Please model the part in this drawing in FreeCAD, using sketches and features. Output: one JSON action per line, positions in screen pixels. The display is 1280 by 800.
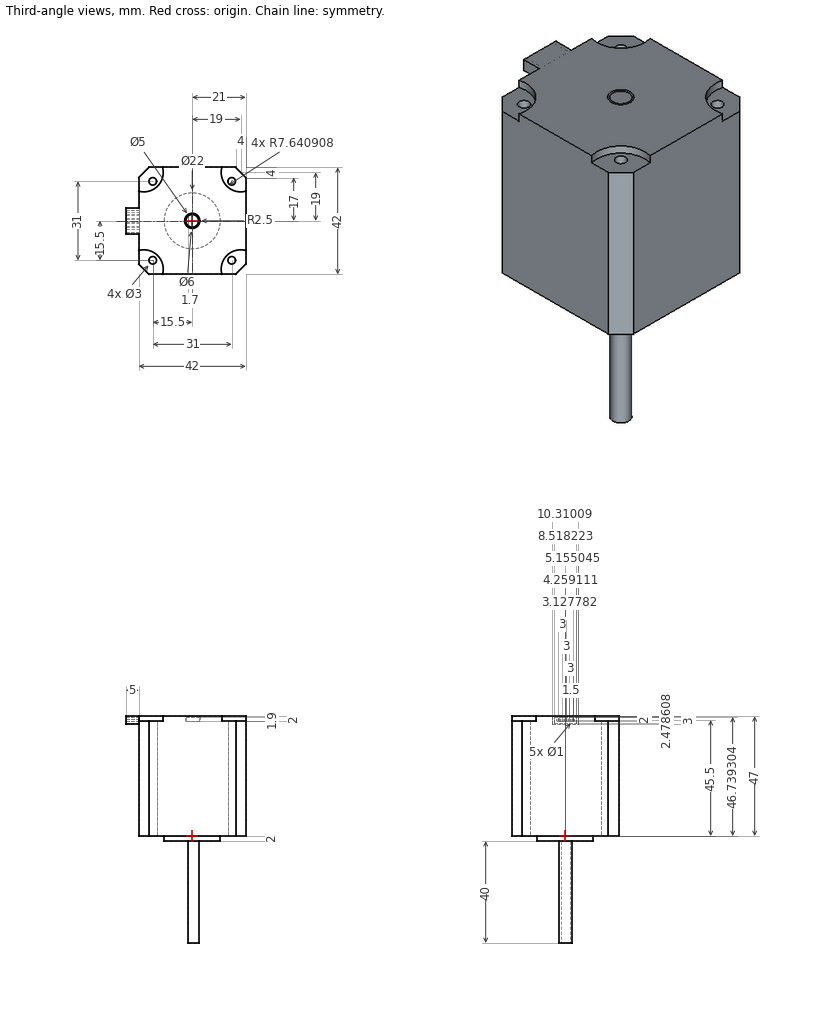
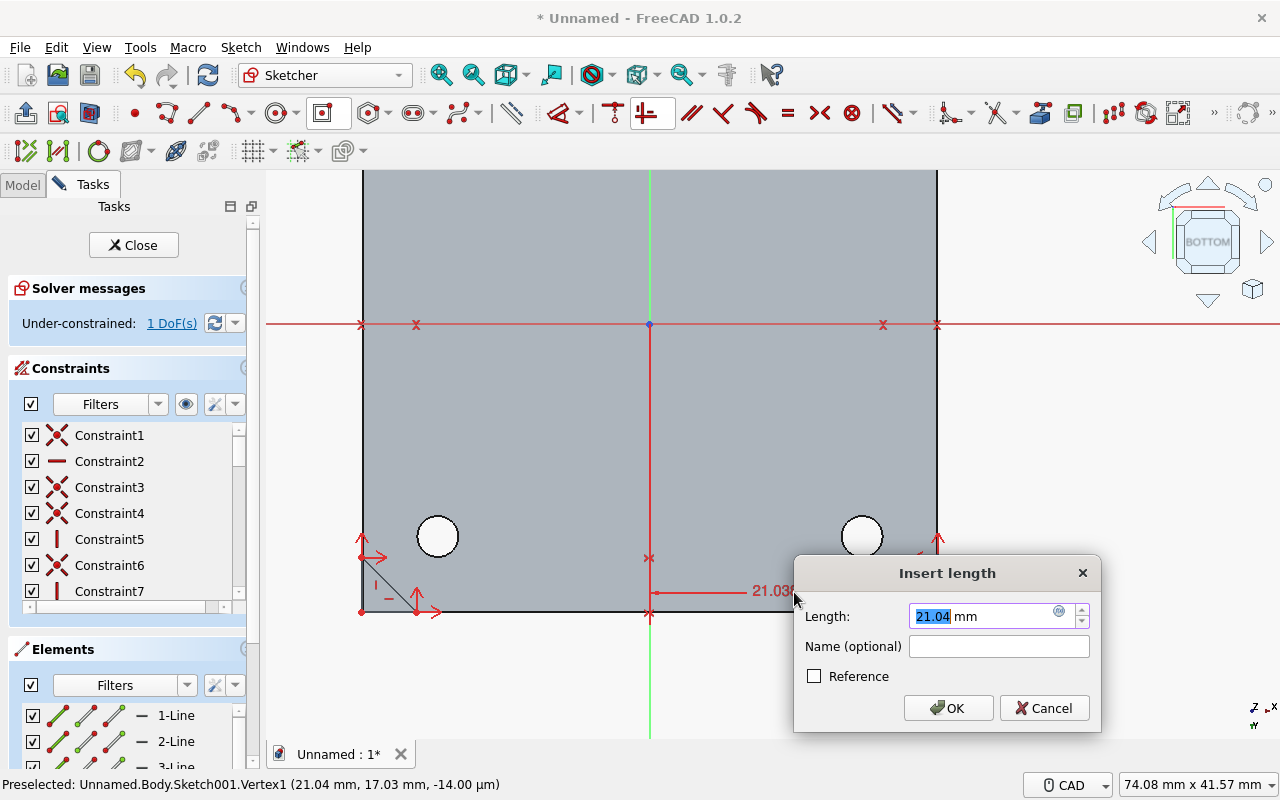
{"action": "type", "text": "21"}
{"action": "key", "text": "Return"}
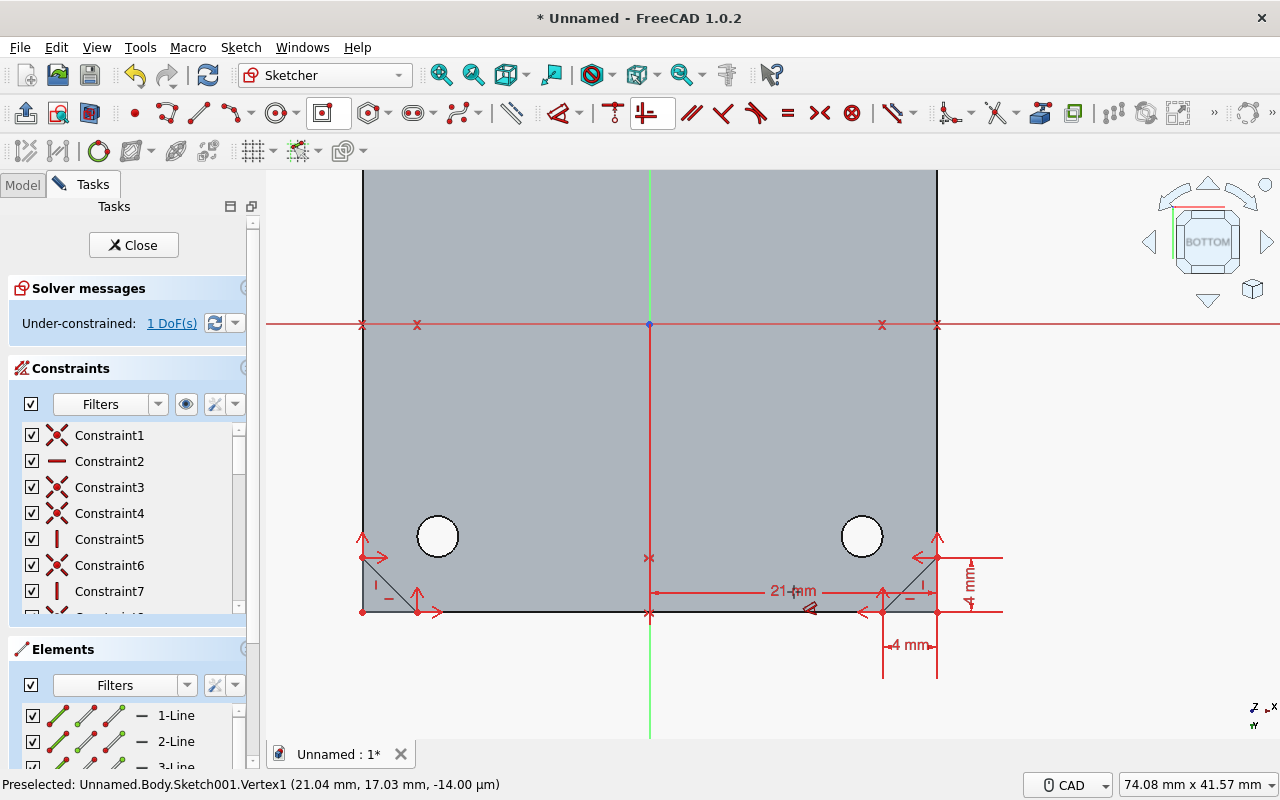
{"action": "left_click", "coordinate": [937, 558]}
{"action": "left_click", "coordinate": [971, 441]}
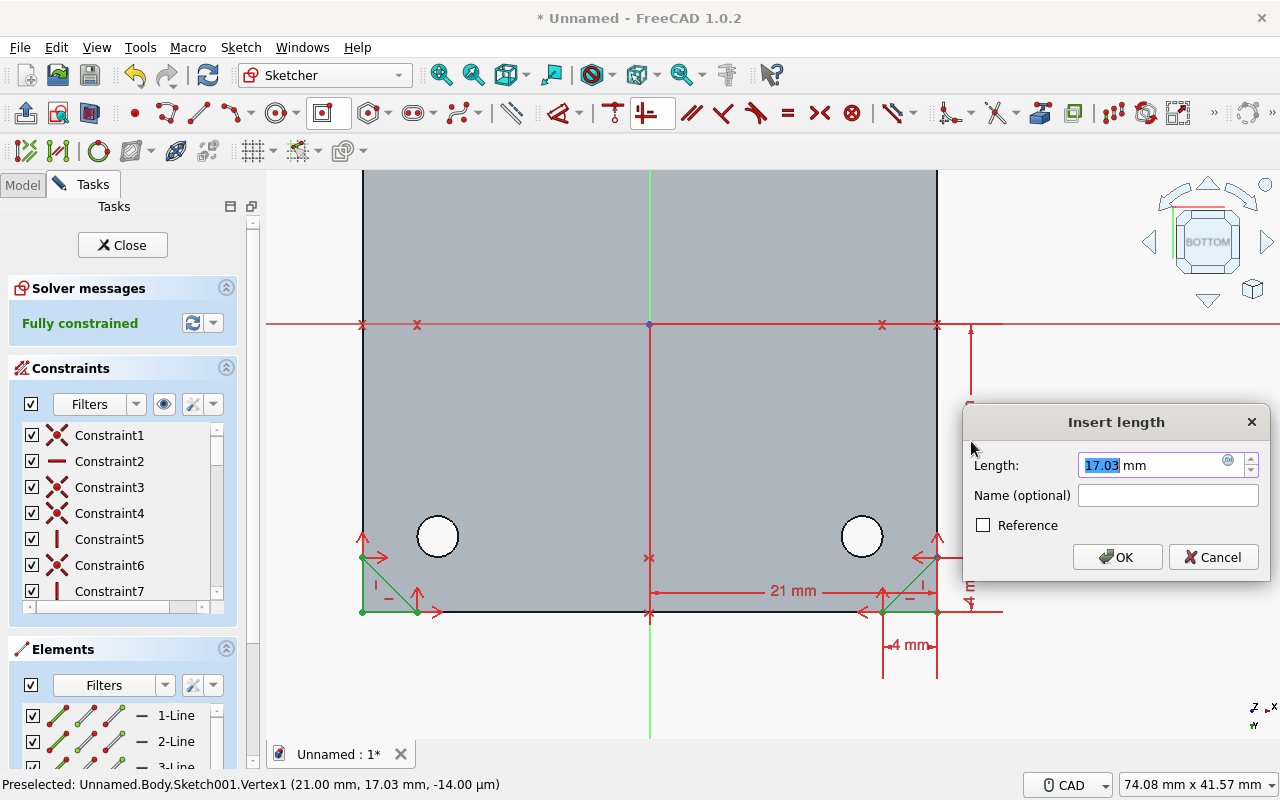
{"action": "type", "text": "17"}
{"action": "key", "text": "Return"}
{"action": "key", "text": "Escape"}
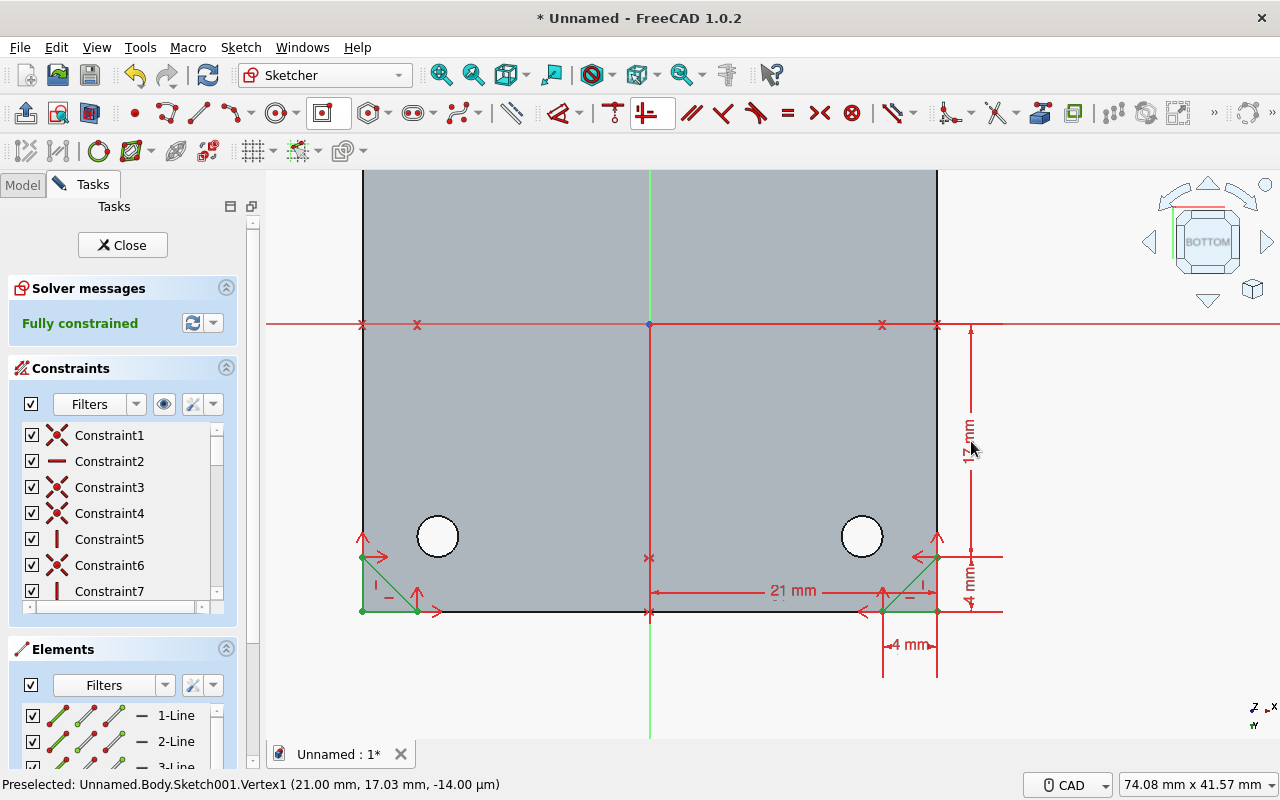
{"action": "left_click", "coordinate": [123, 245]}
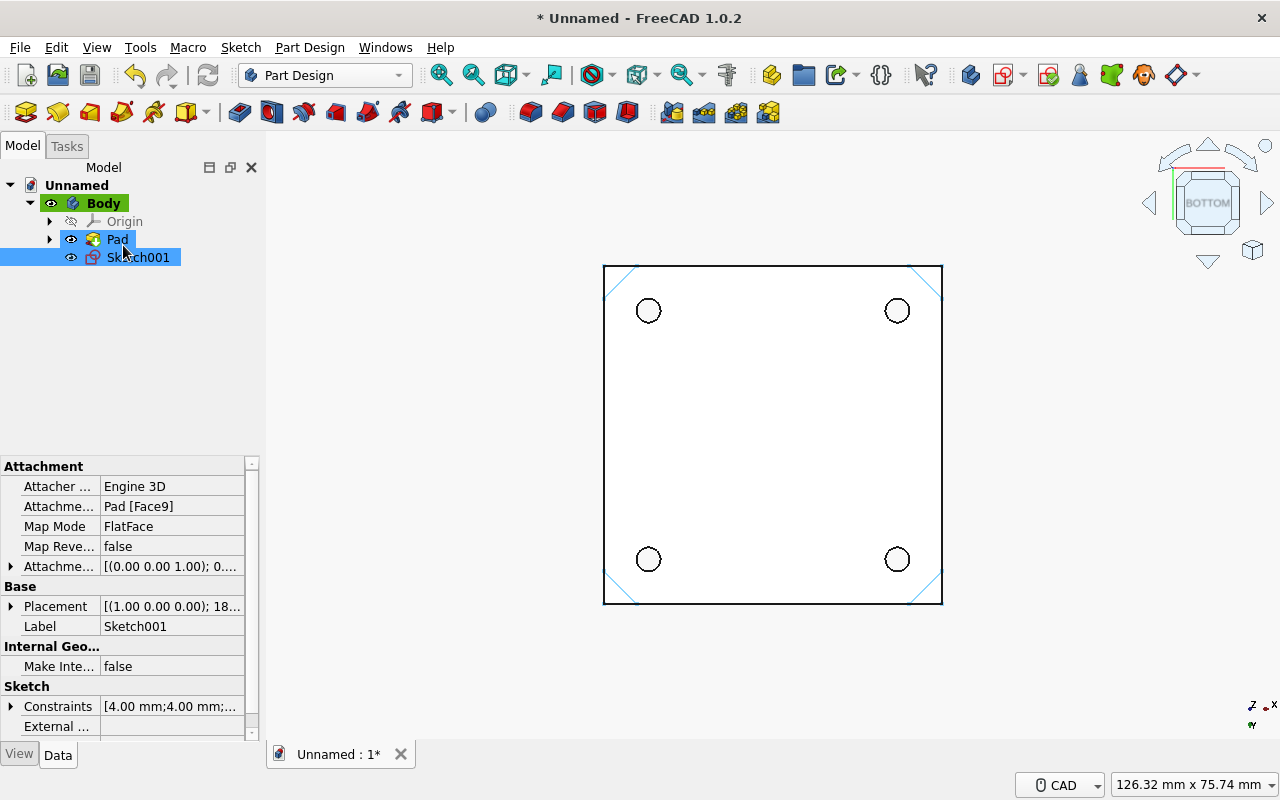
{"action": "left_click", "coordinate": [240, 112]}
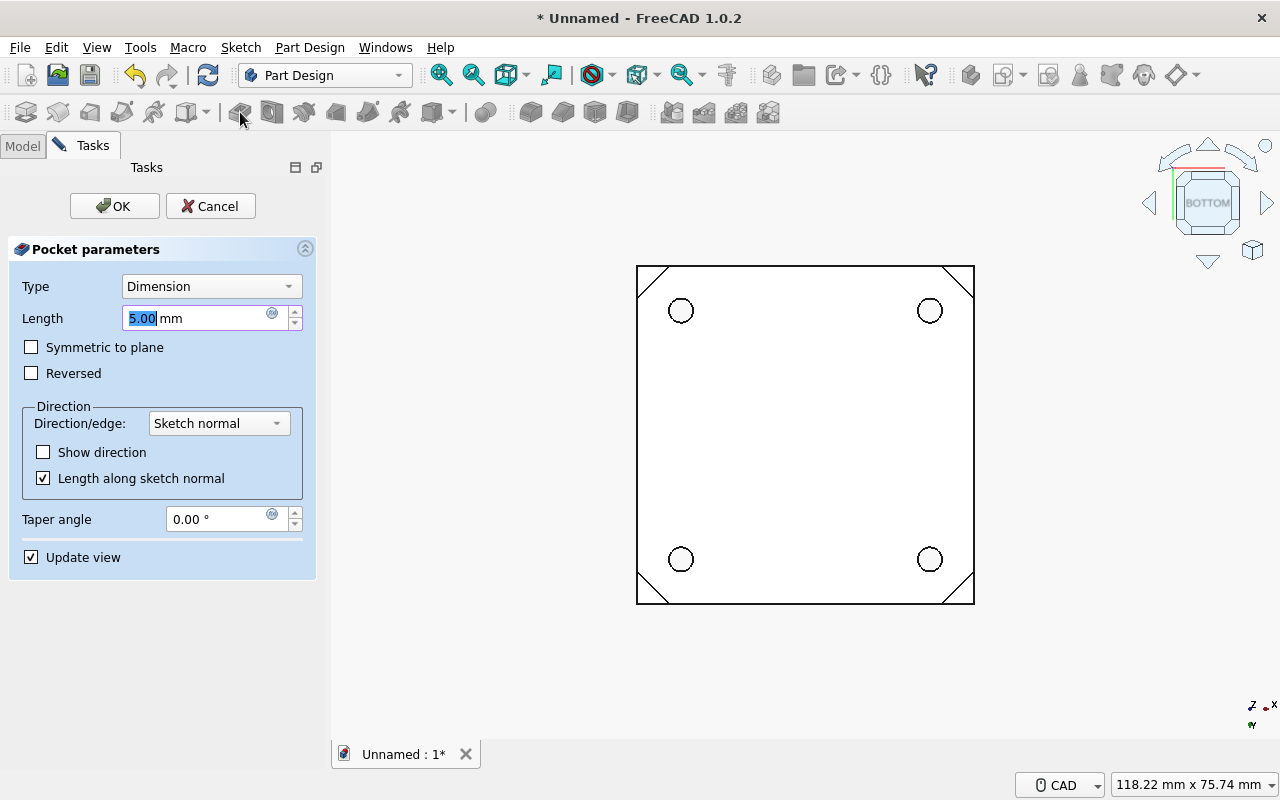
{"action": "left_click", "coordinate": [212, 286]}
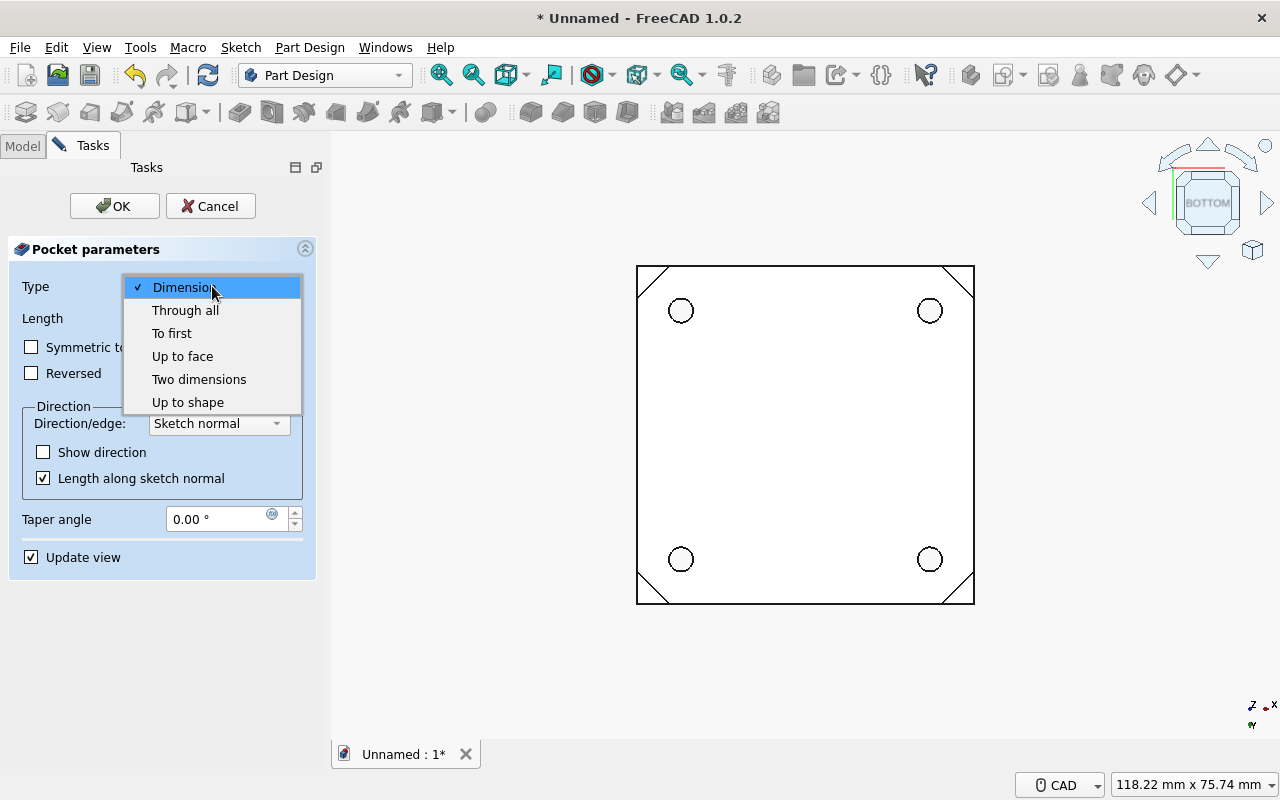
{"action": "left_click", "coordinate": [212, 310]}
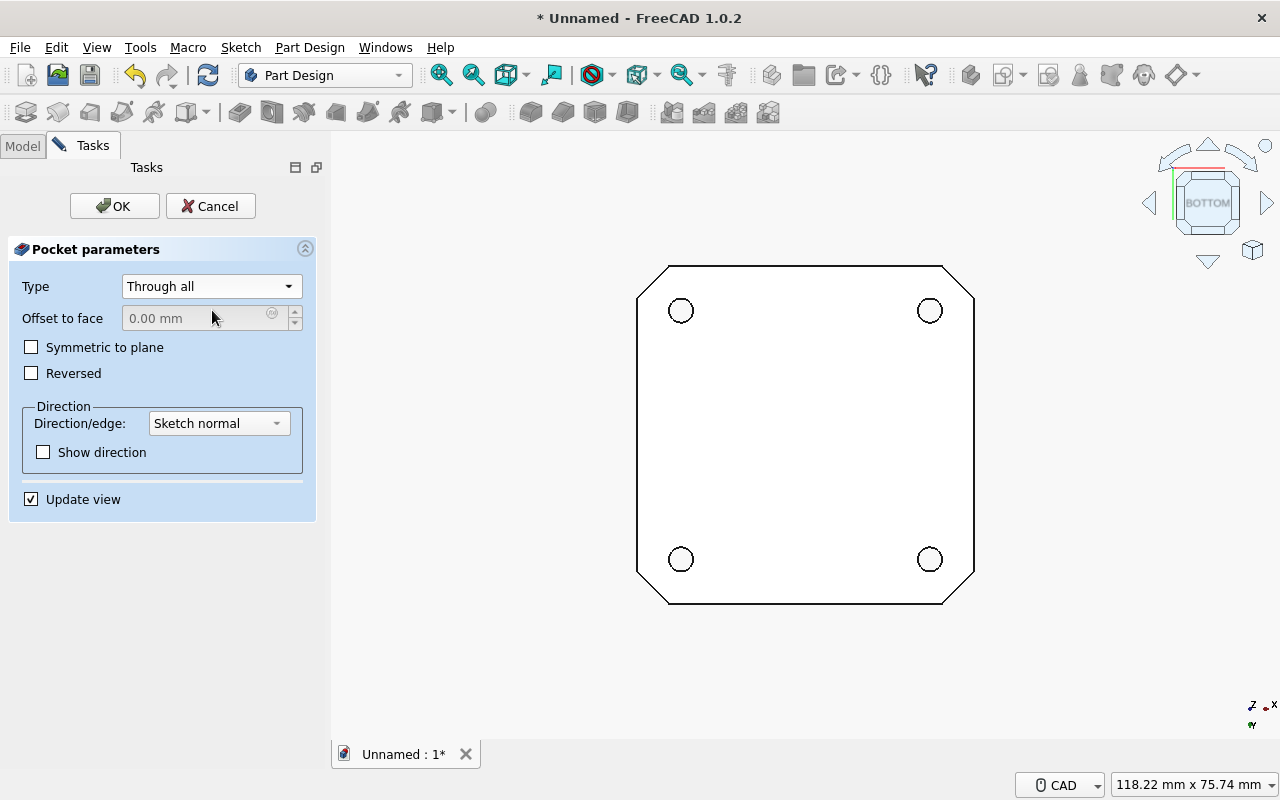
{"action": "left_click", "coordinate": [115, 206]}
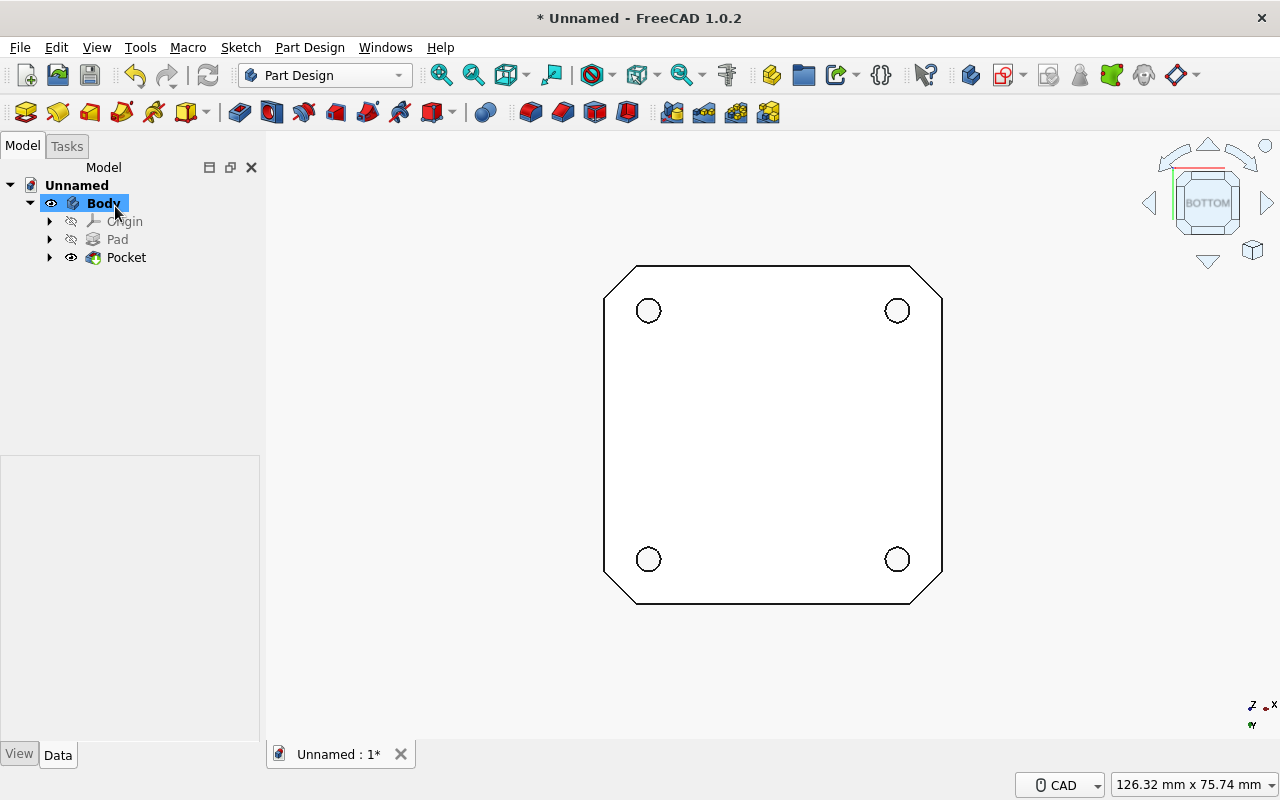
{"action": "left_click", "coordinate": [773, 434]}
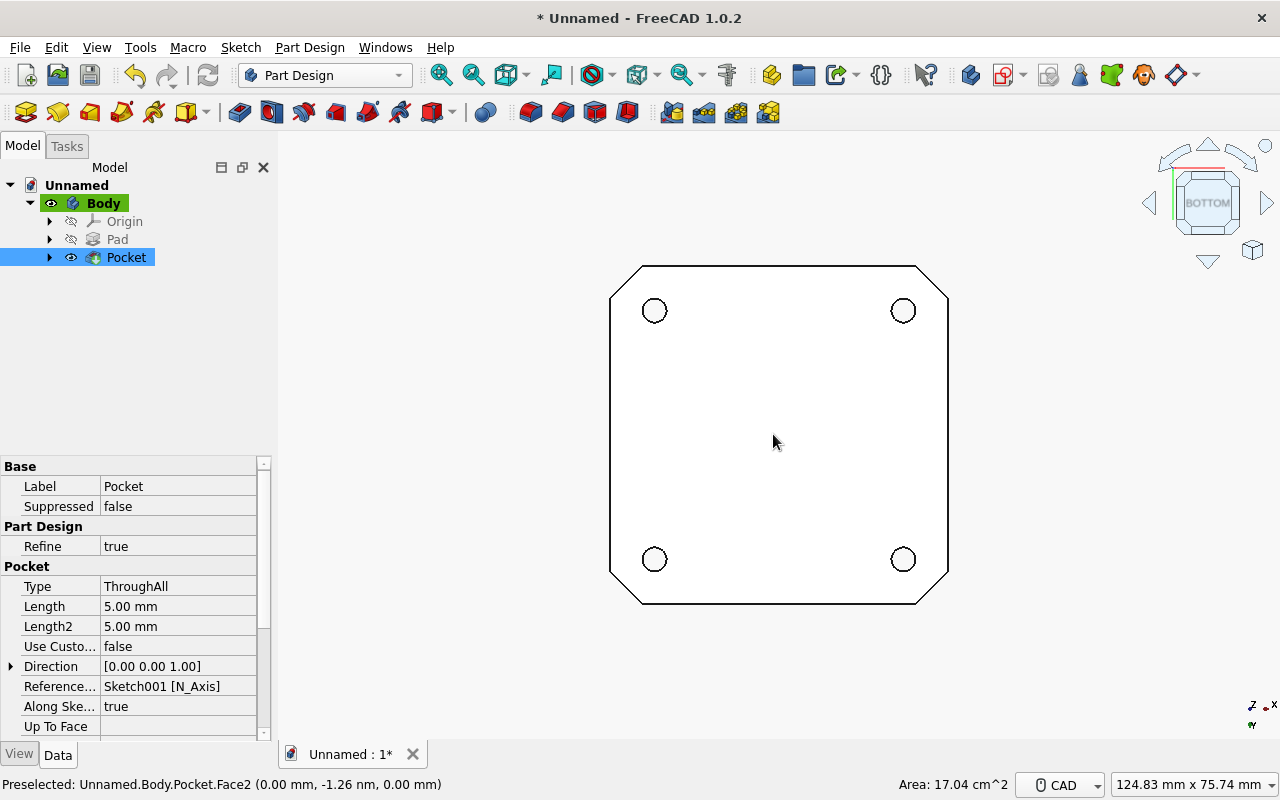
{"action": "left_click", "coordinate": [1004, 76]}